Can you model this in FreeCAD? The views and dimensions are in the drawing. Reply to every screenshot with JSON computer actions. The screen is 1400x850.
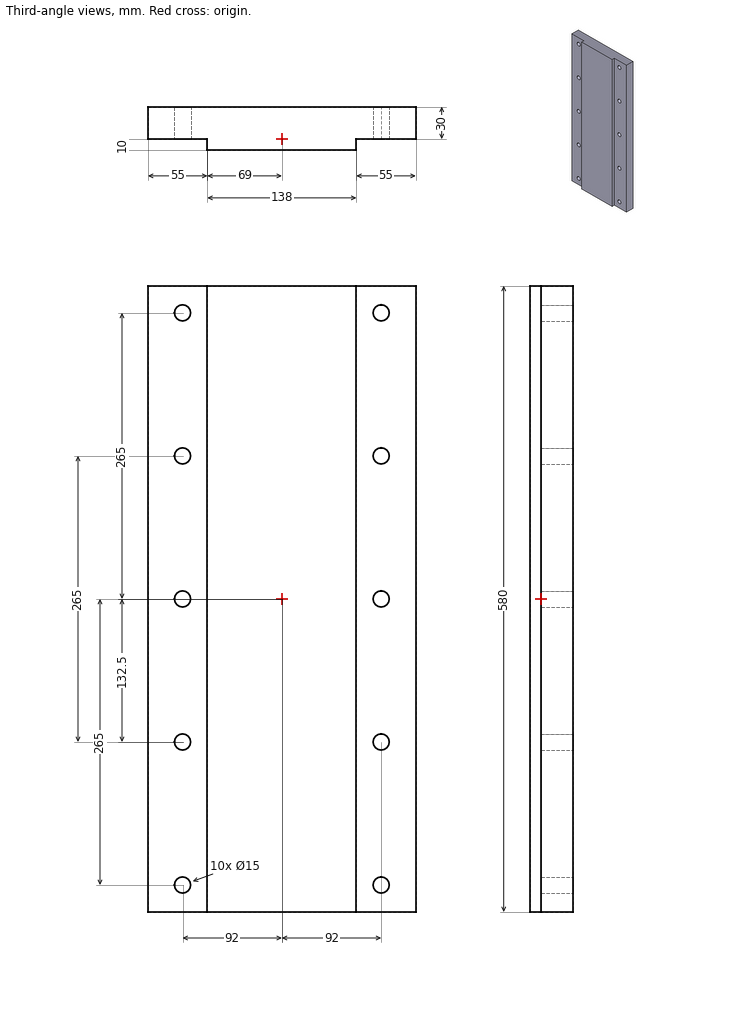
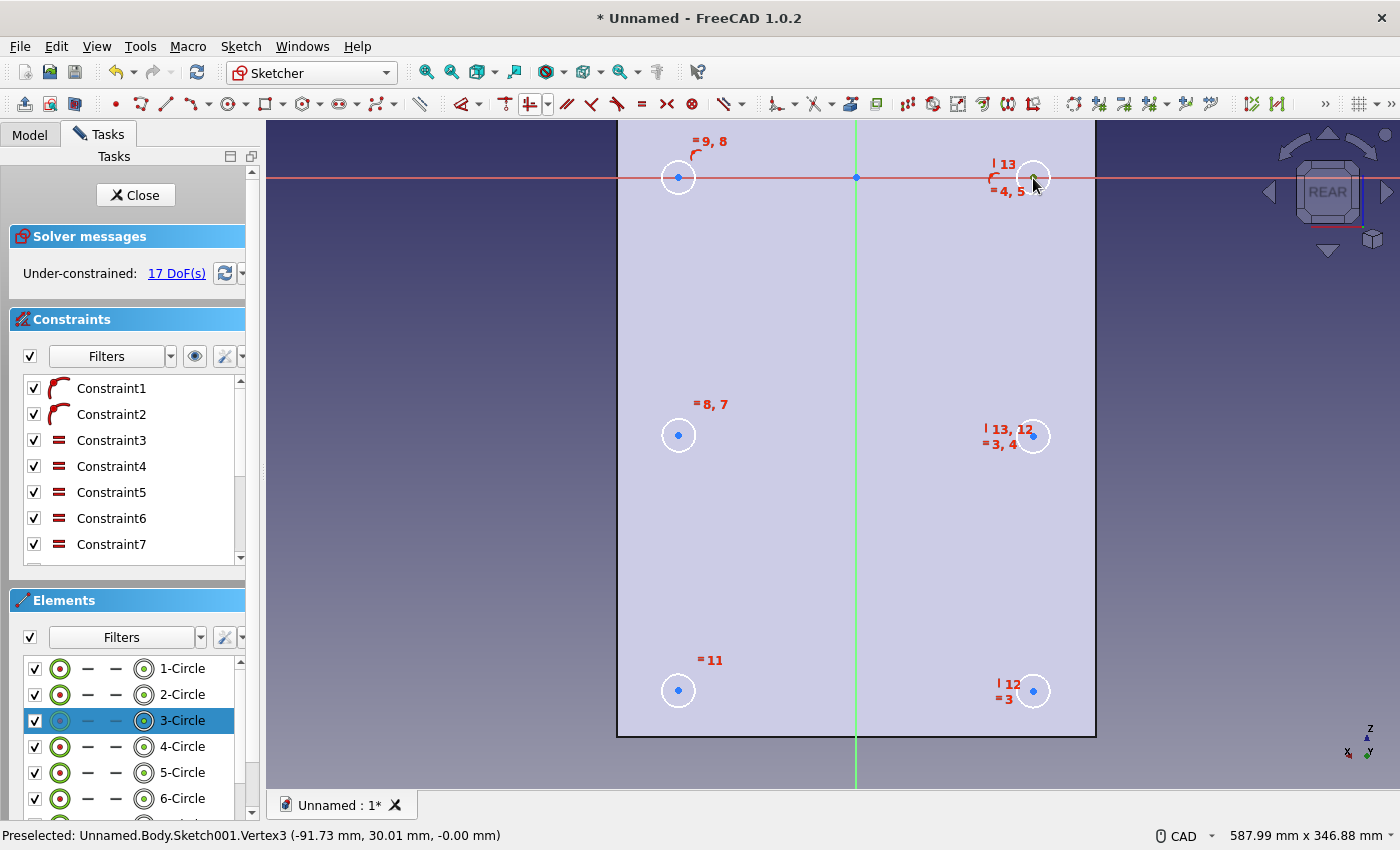
{"action": "scroll", "coordinate": [690, 680], "scroll_direction": "down", "scroll_amount": 4}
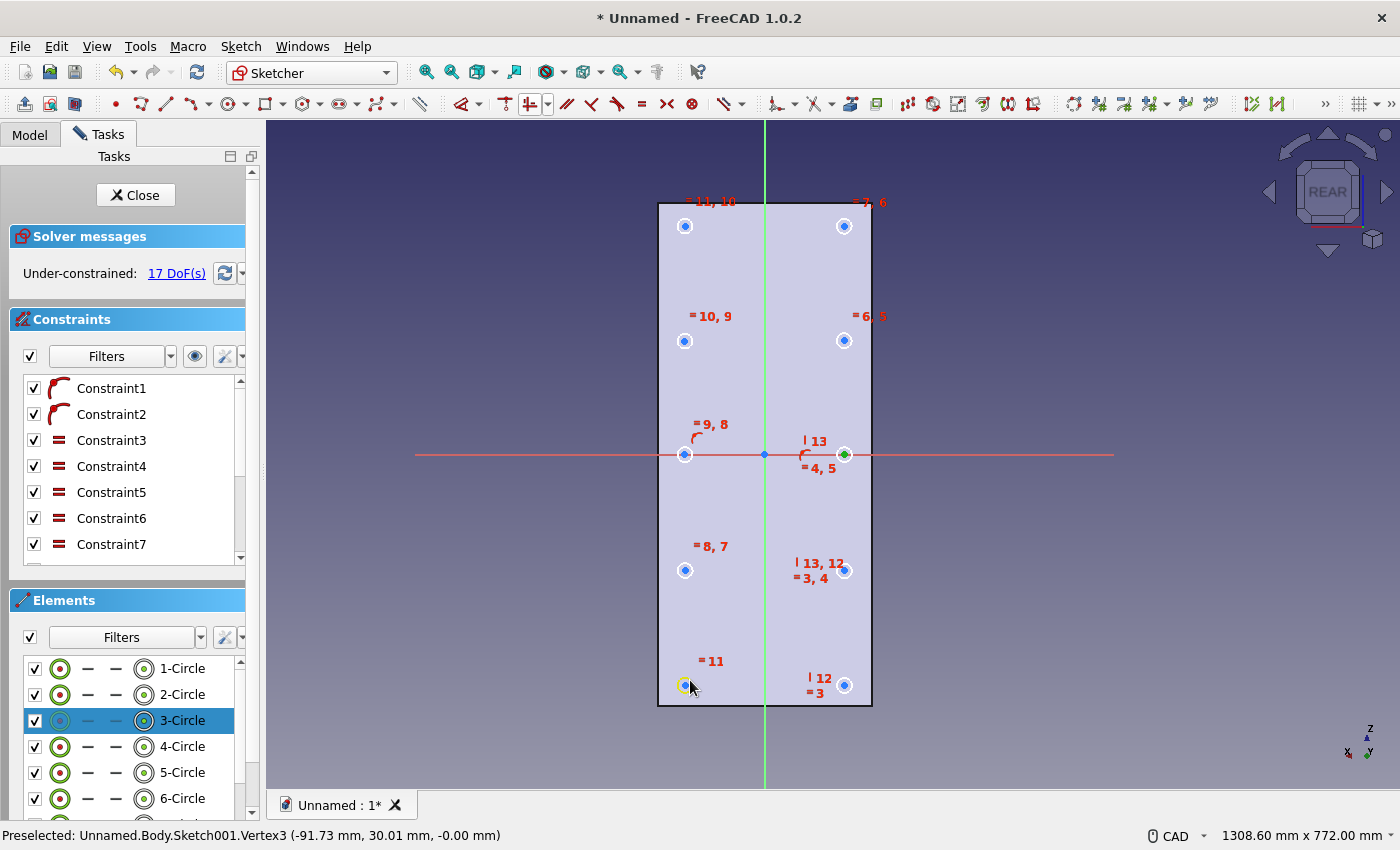
{"action": "left_click", "coordinate": [844, 341]}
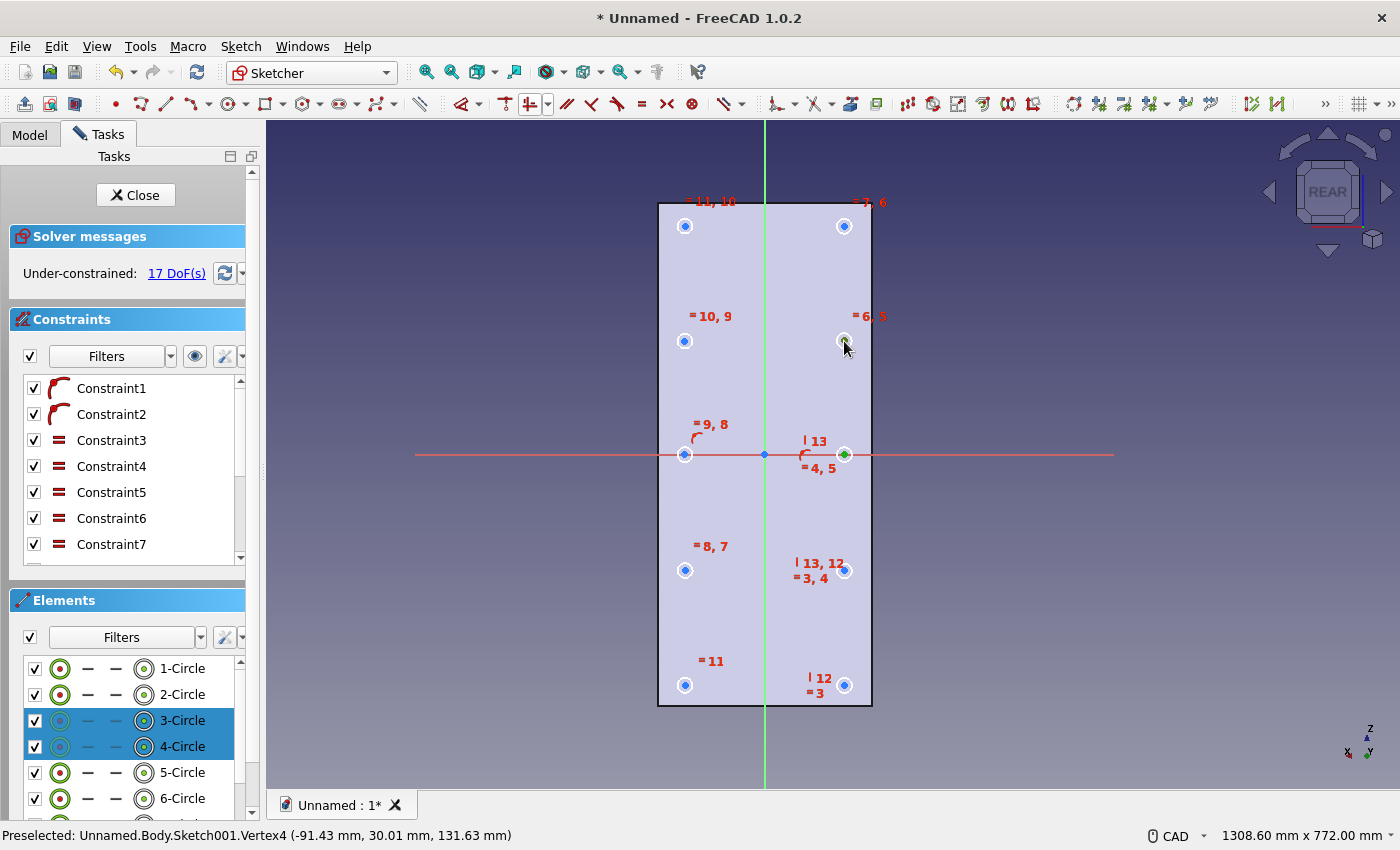
{"action": "left_click", "coordinate": [548, 104]}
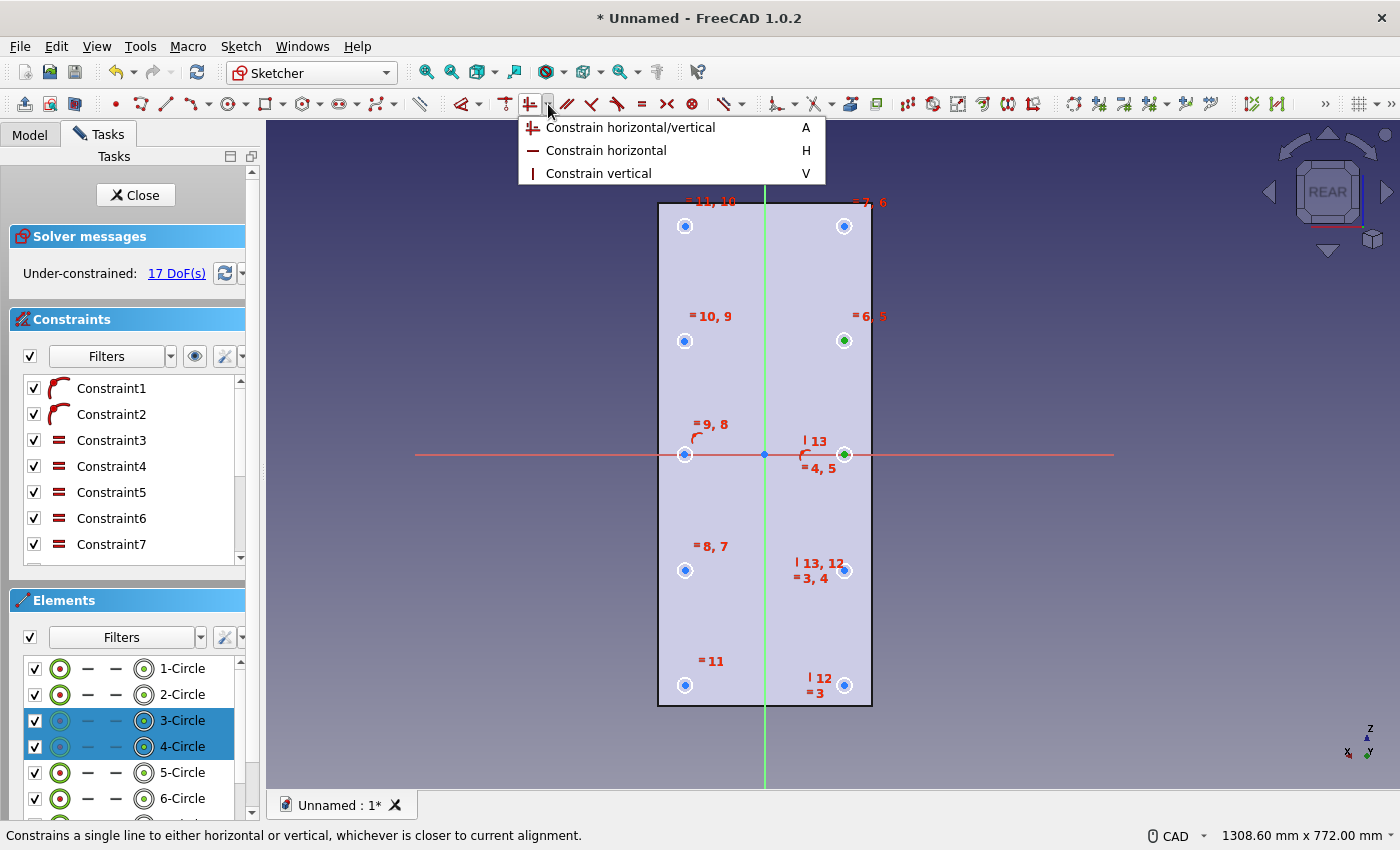
{"action": "left_click", "coordinate": [672, 174]}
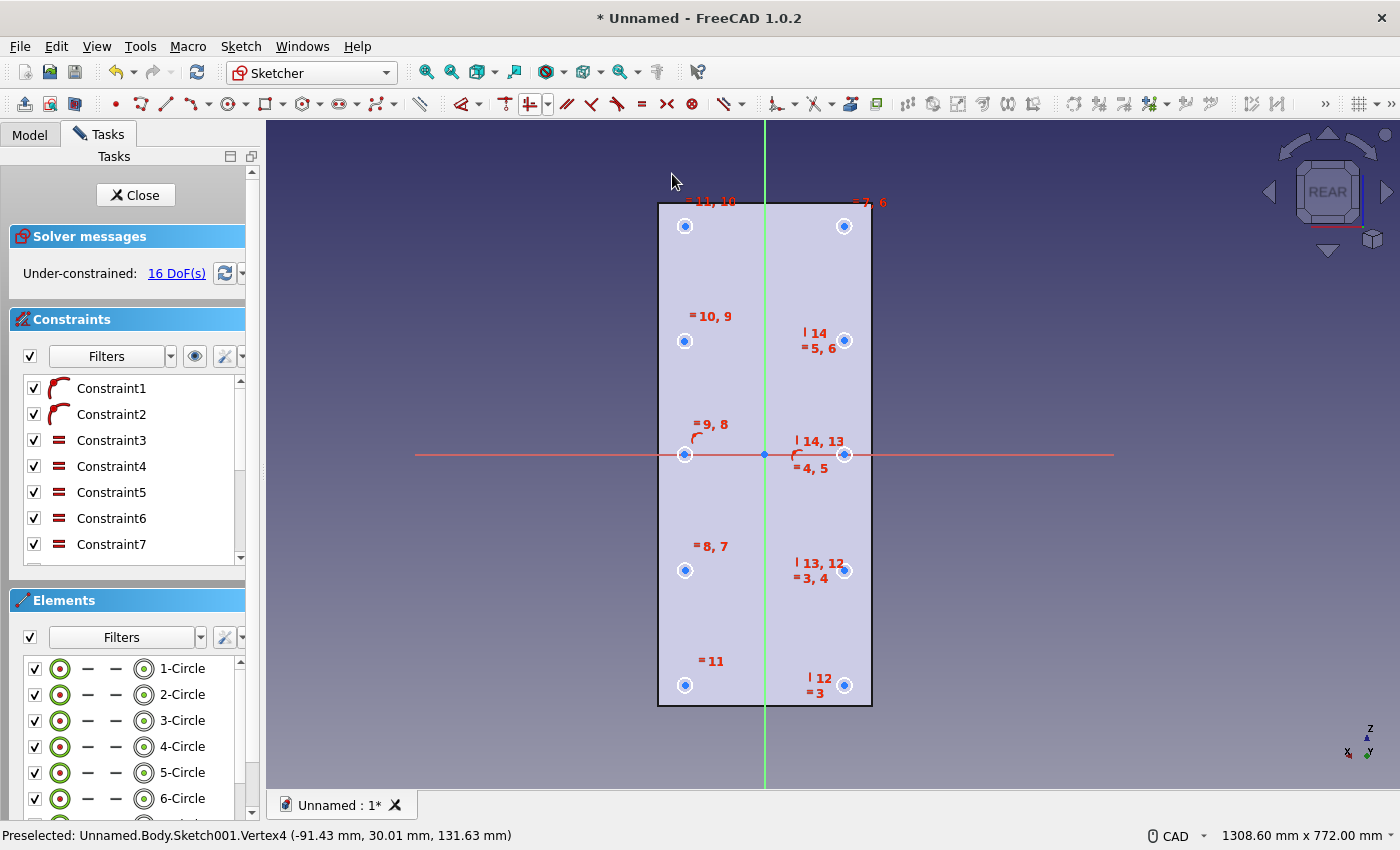
{"action": "left_click", "coordinate": [844, 341]}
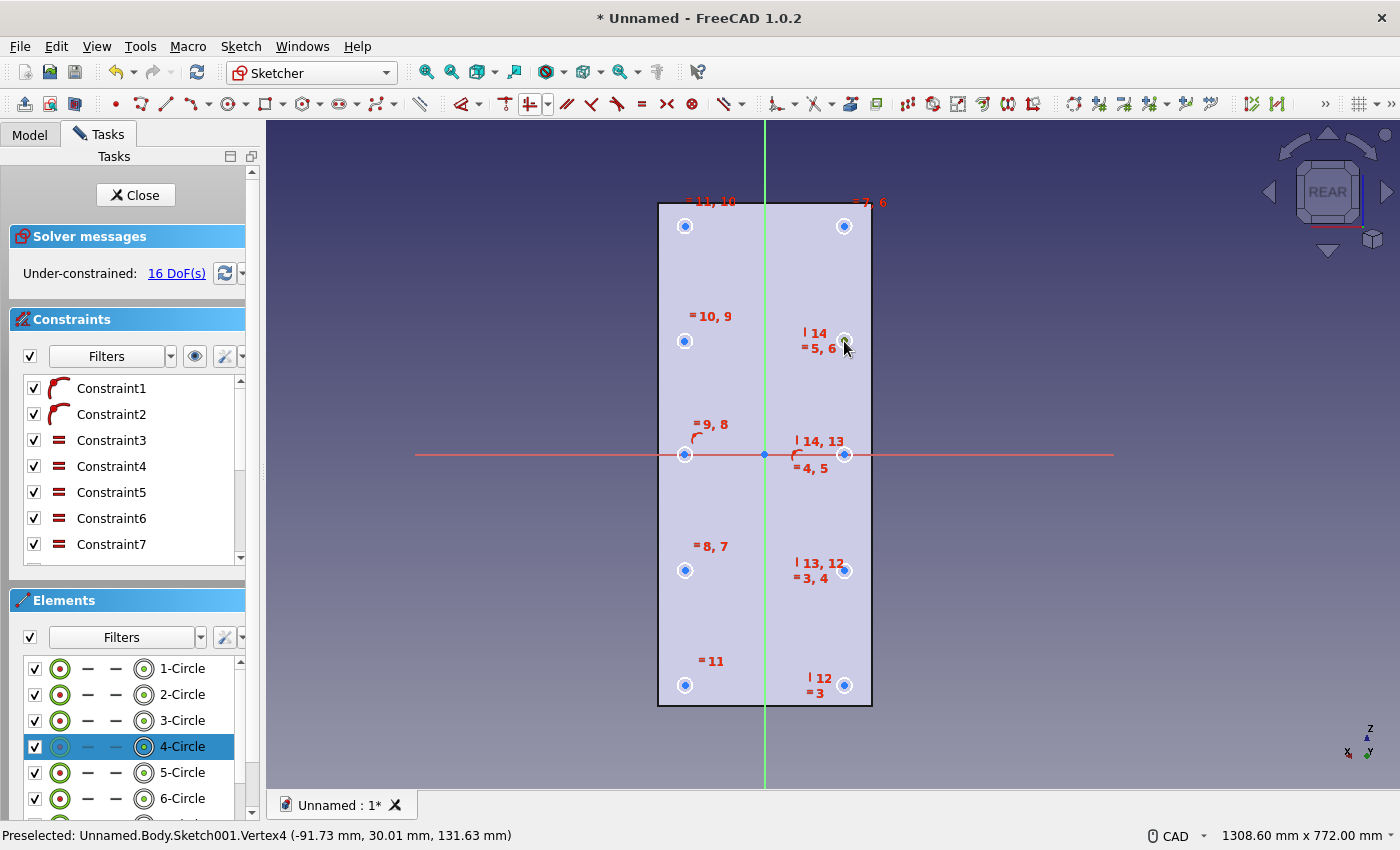
{"action": "left_click", "coordinate": [844, 226]}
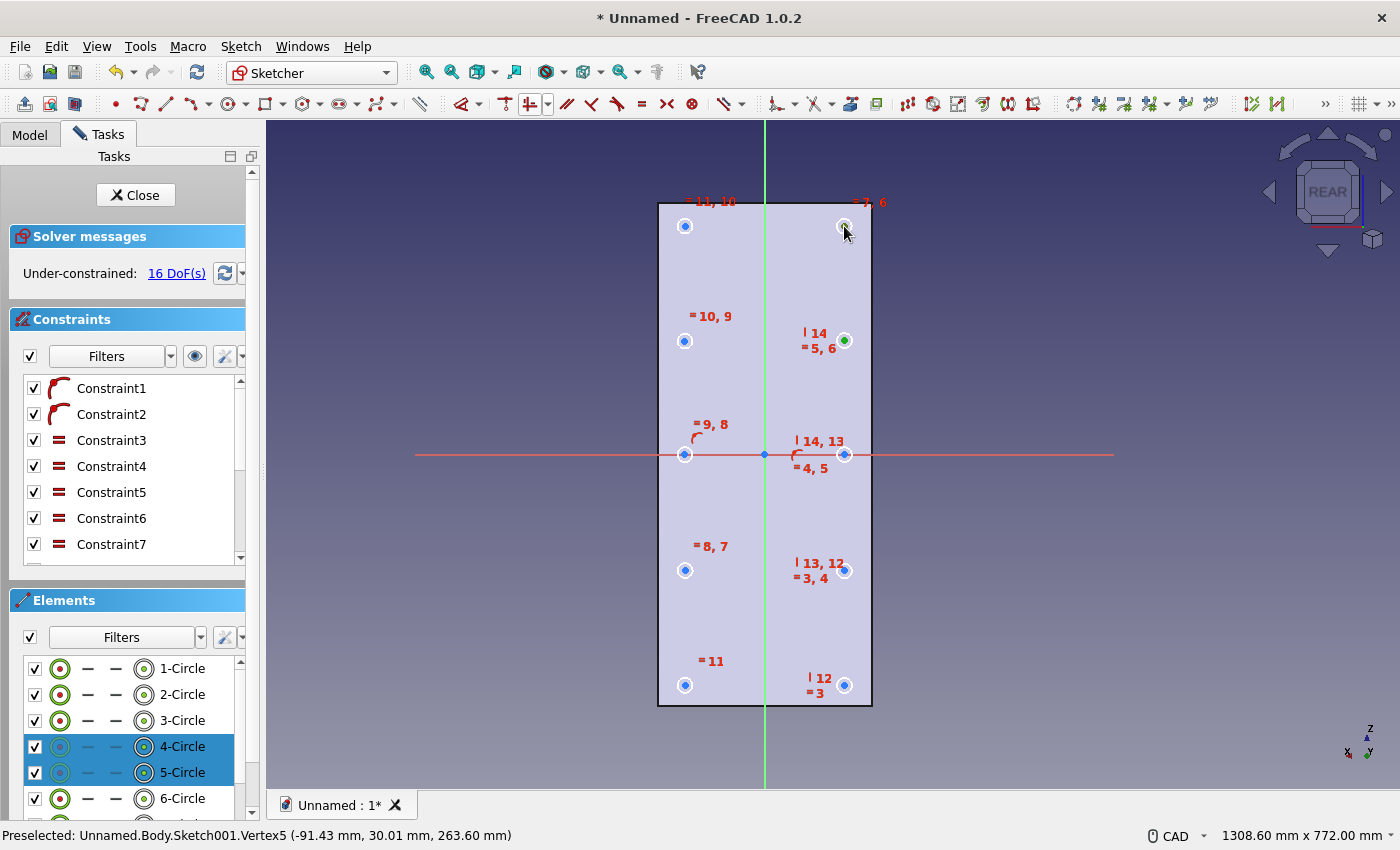
{"action": "left_click", "coordinate": [548, 104]}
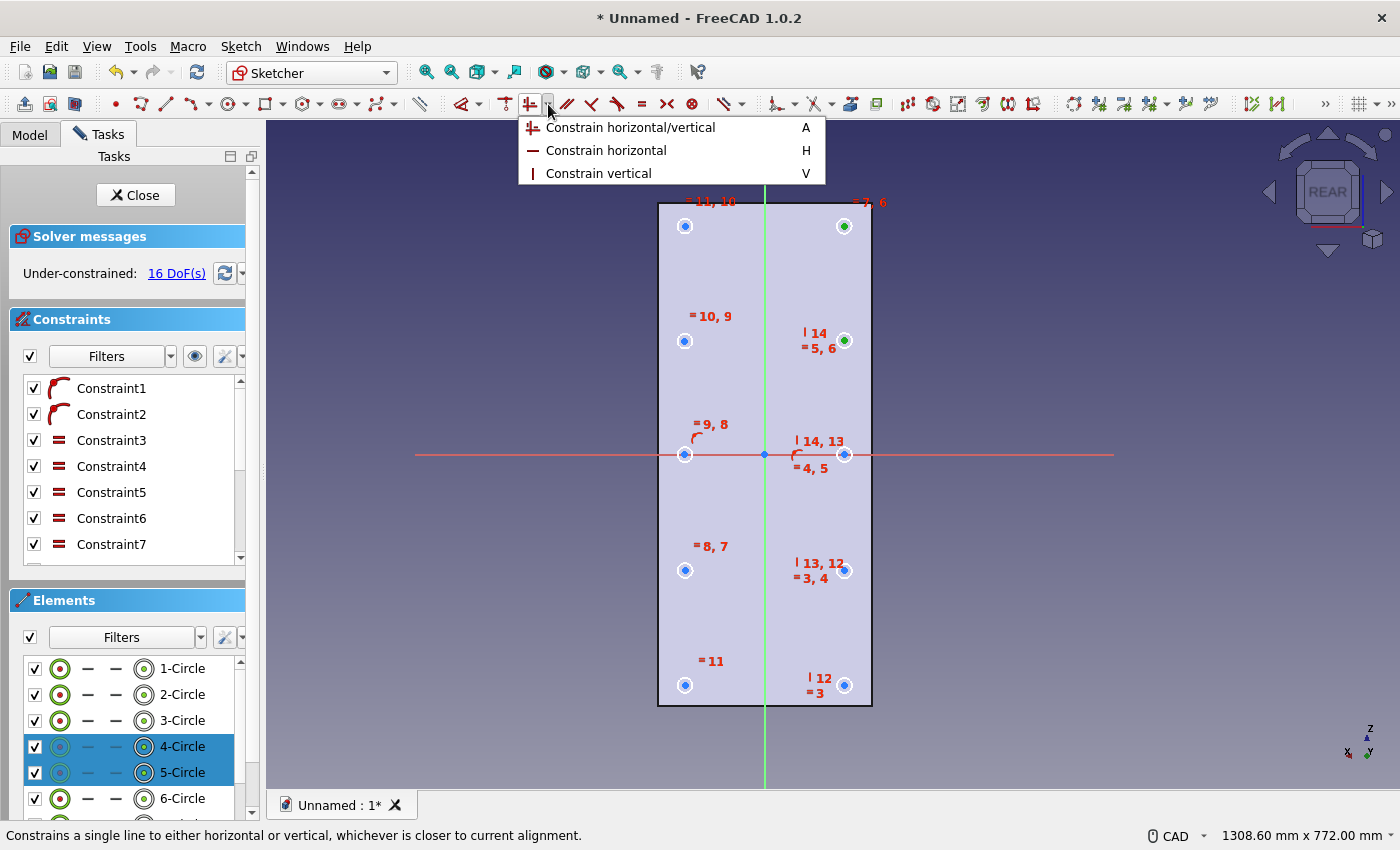
{"action": "left_click", "coordinate": [672, 174]}